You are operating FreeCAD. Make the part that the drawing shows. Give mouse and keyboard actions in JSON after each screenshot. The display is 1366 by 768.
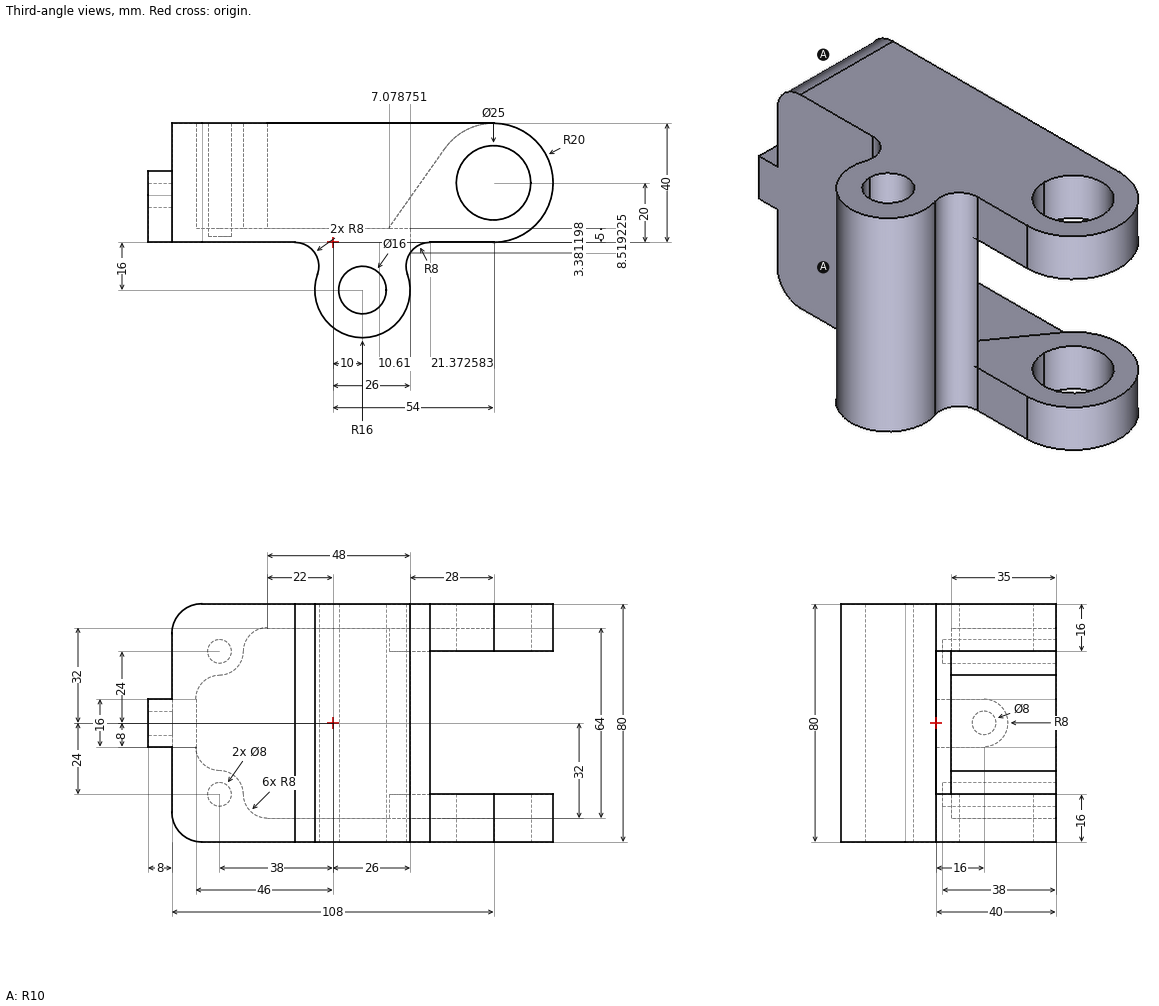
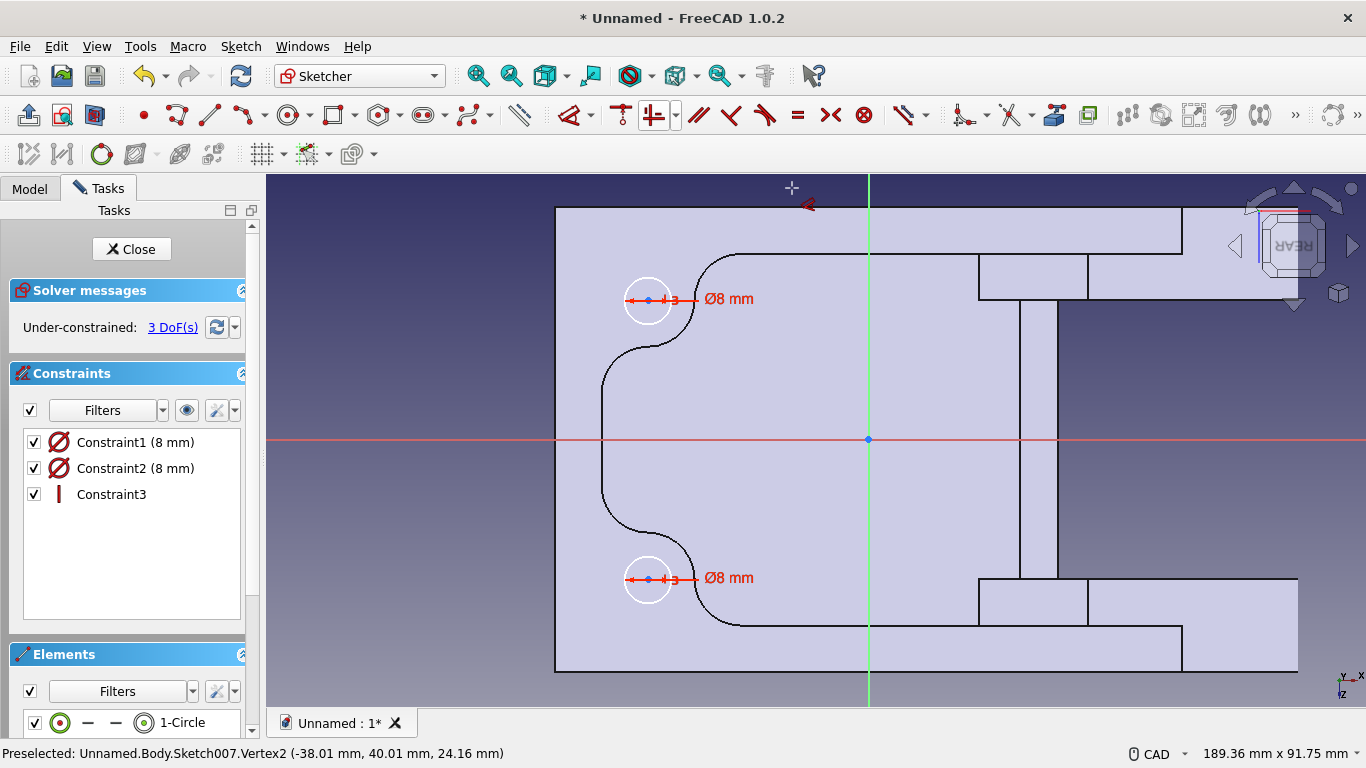
{"action": "left_click", "coordinate": [648, 301]}
{"action": "left_click", "coordinate": [758, 267]}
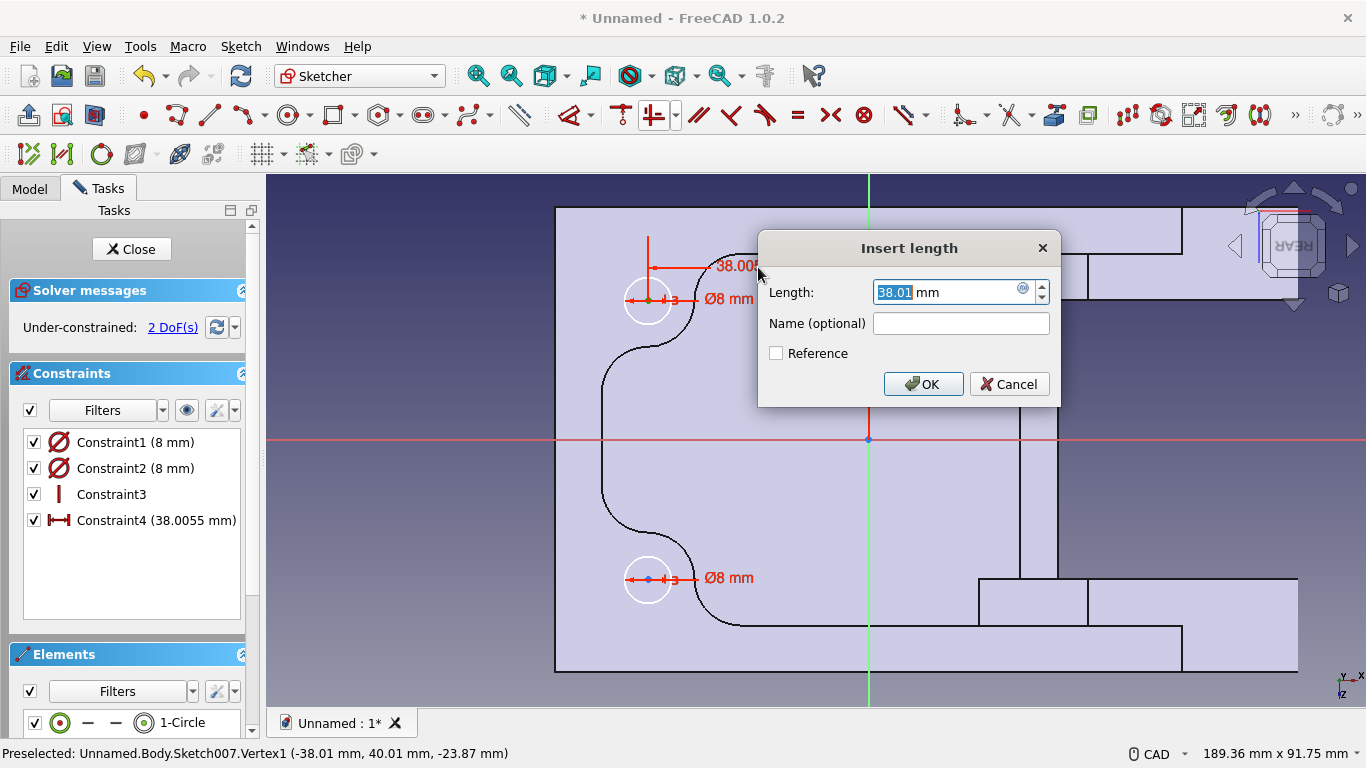
{"action": "type", "text": "38"}
{"action": "key", "text": "Return"}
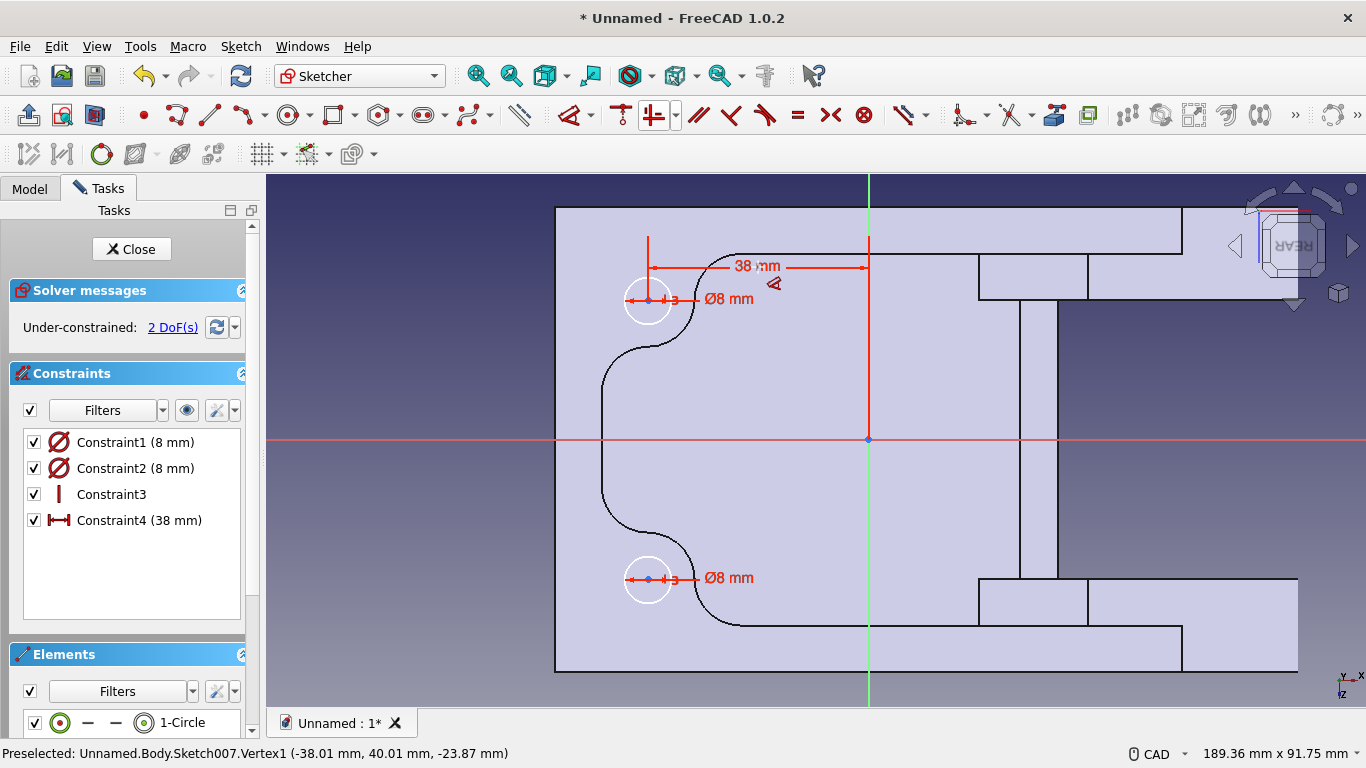
{"action": "left_click", "coordinate": [648, 301]}
{"action": "left_click", "coordinate": [903, 370]}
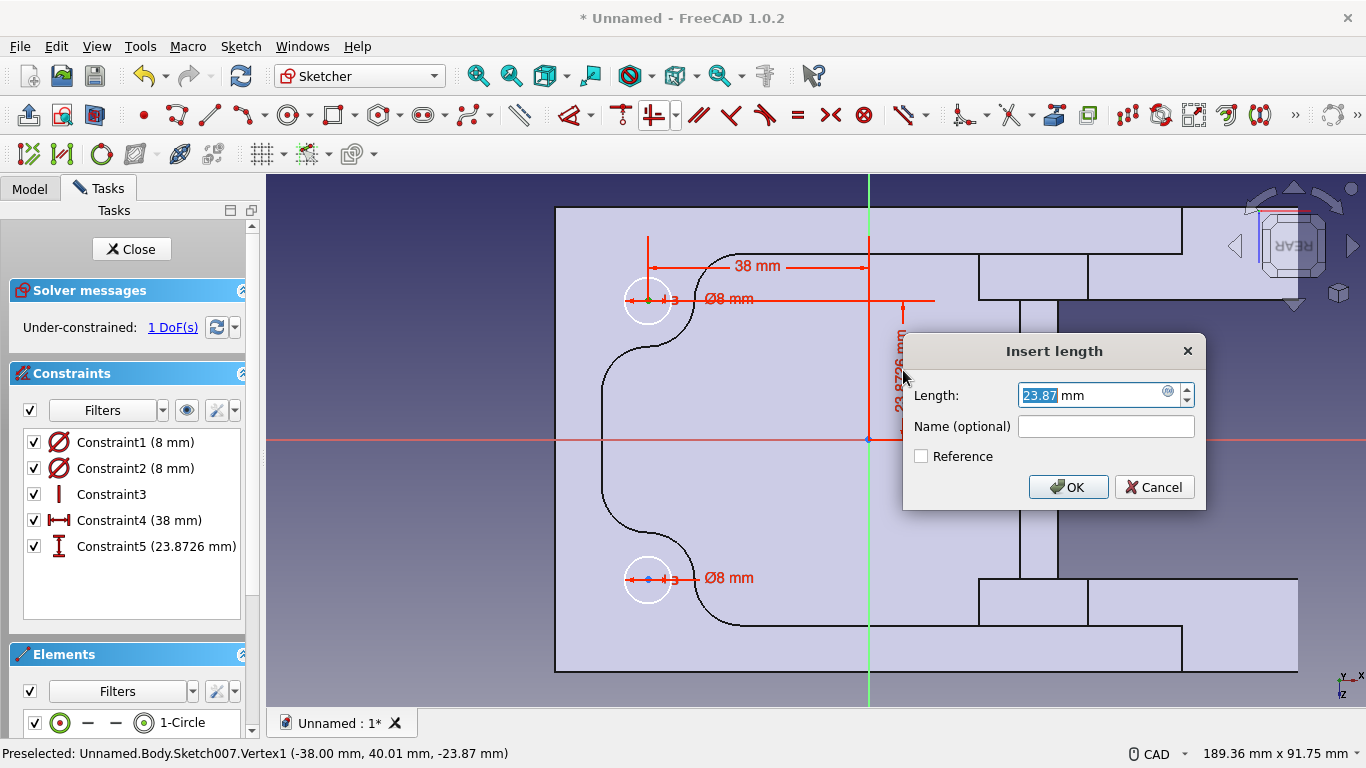
{"action": "type", "text": "24"}
{"action": "key", "text": "Return"}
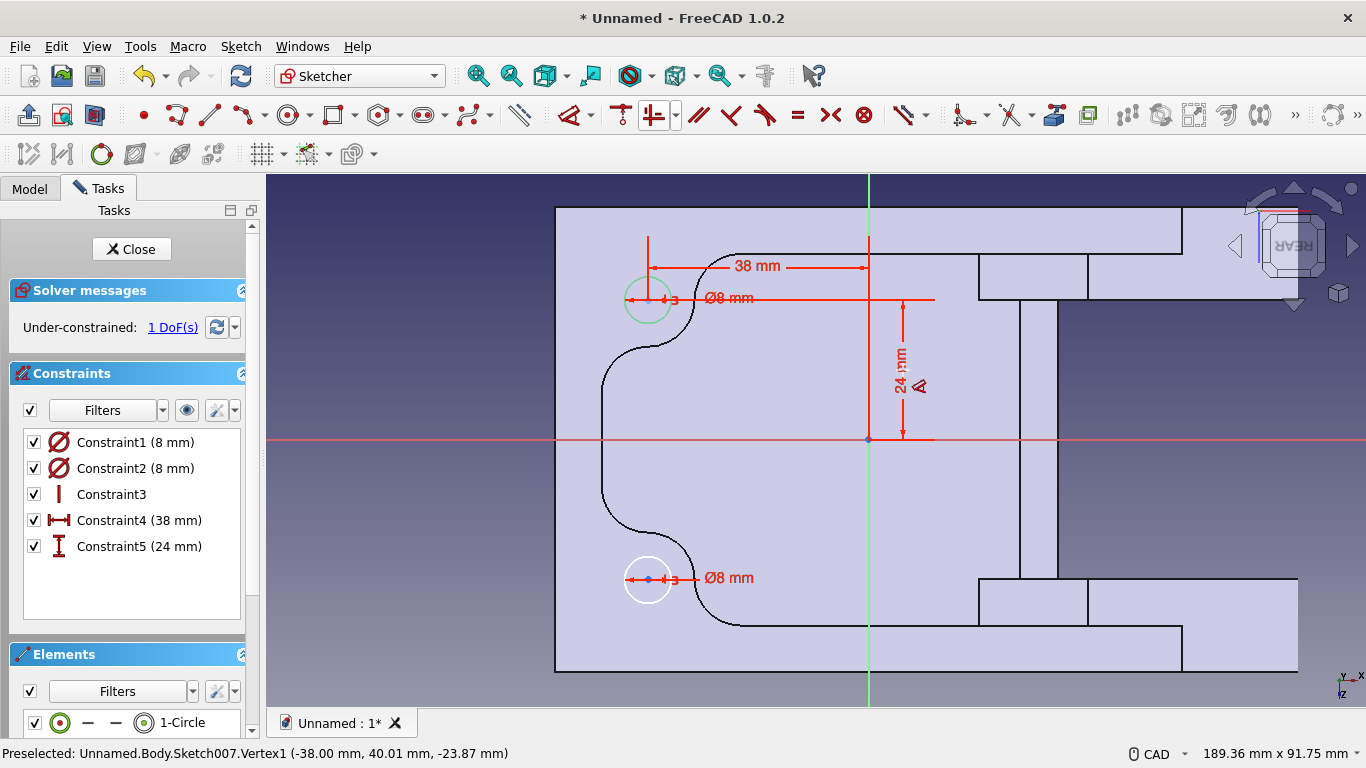
{"action": "left_click", "coordinate": [648, 580]}
{"action": "left_click", "coordinate": [903, 510]}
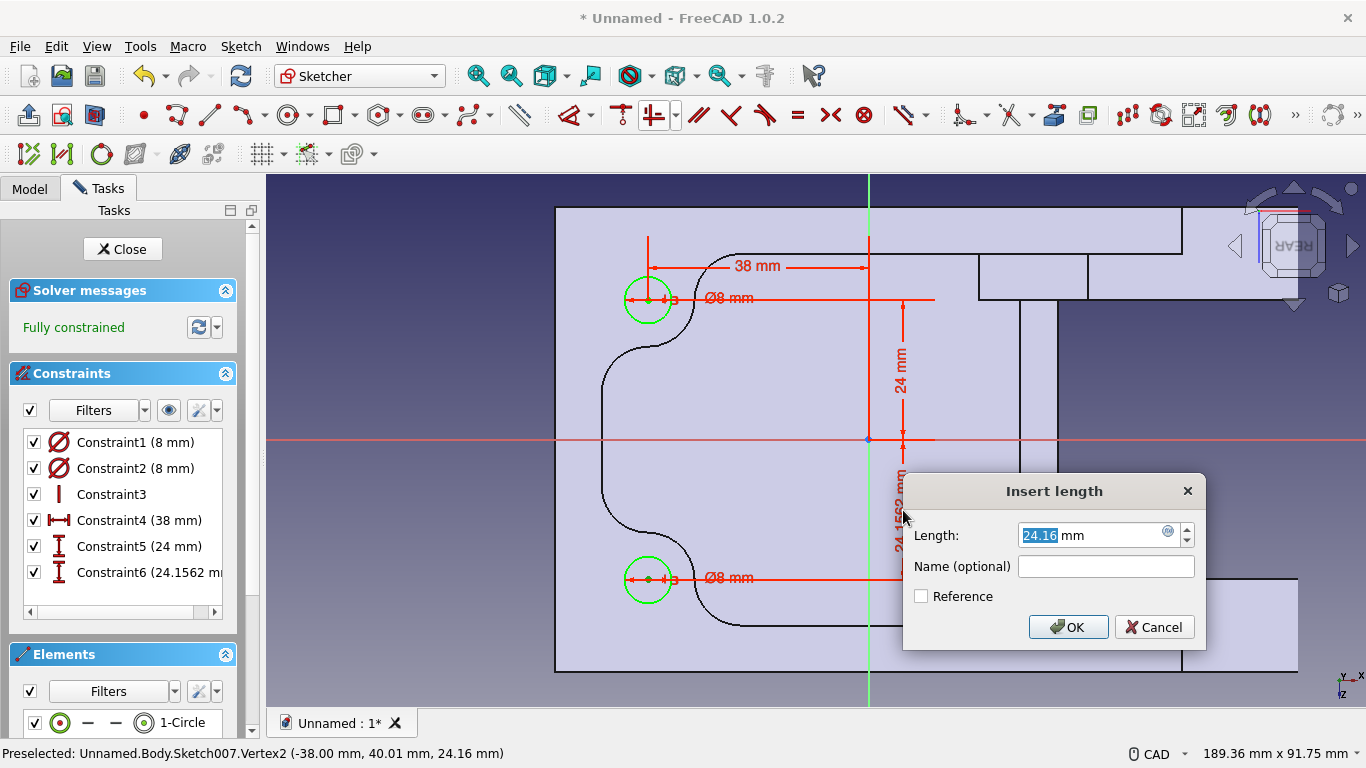
{"action": "type", "text": "24"}
{"action": "key", "text": "Return"}
{"action": "key", "text": "Escape"}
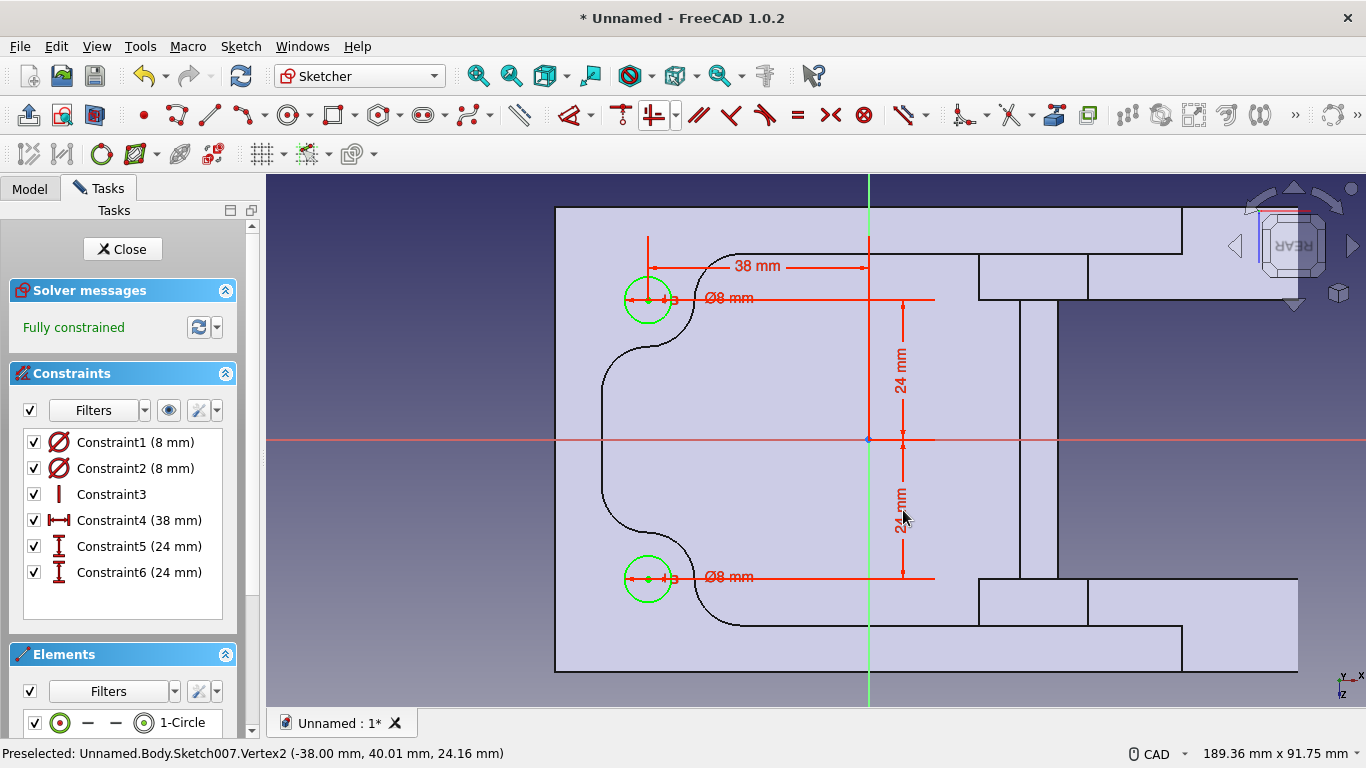
{"action": "left_click", "coordinate": [123, 249]}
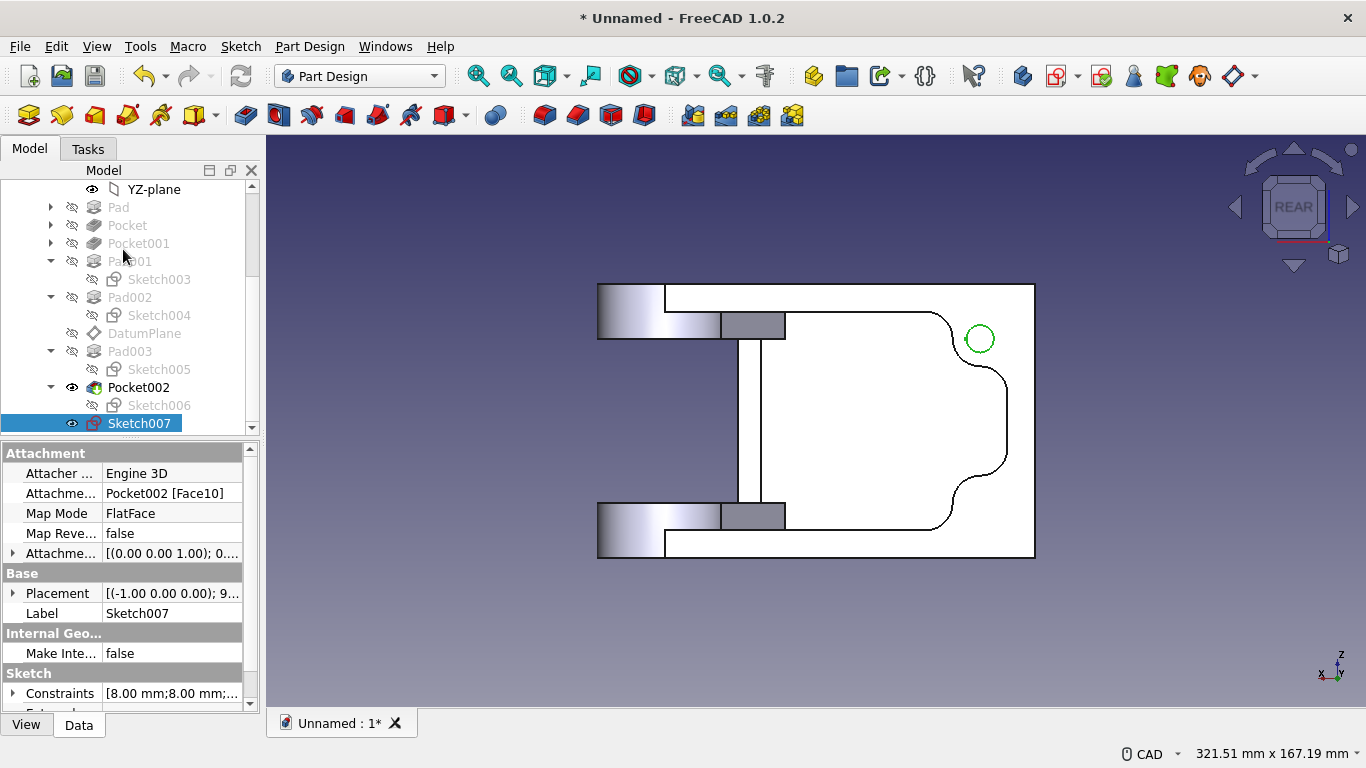
{"action": "left_click", "coordinate": [246, 116]}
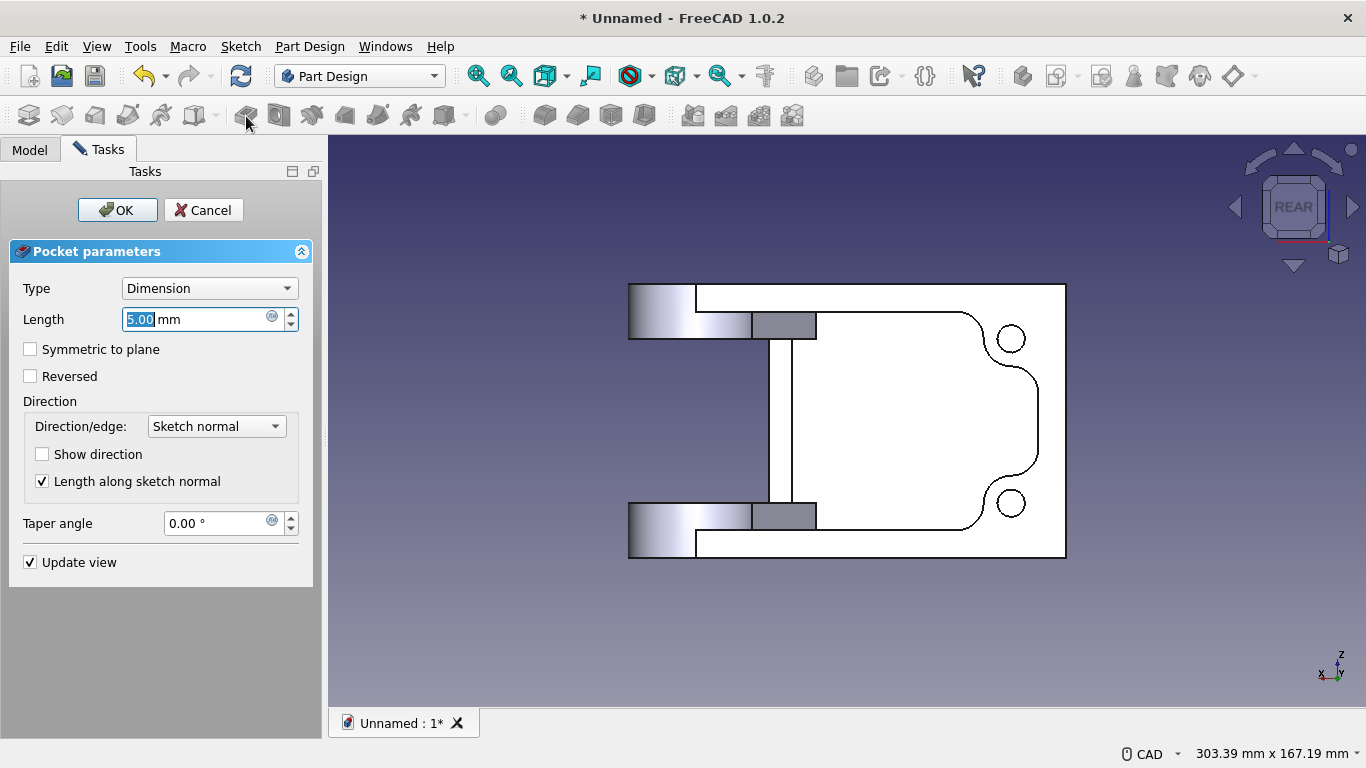
{"action": "type", "text": "38"}
{"action": "key", "text": "Tab"}